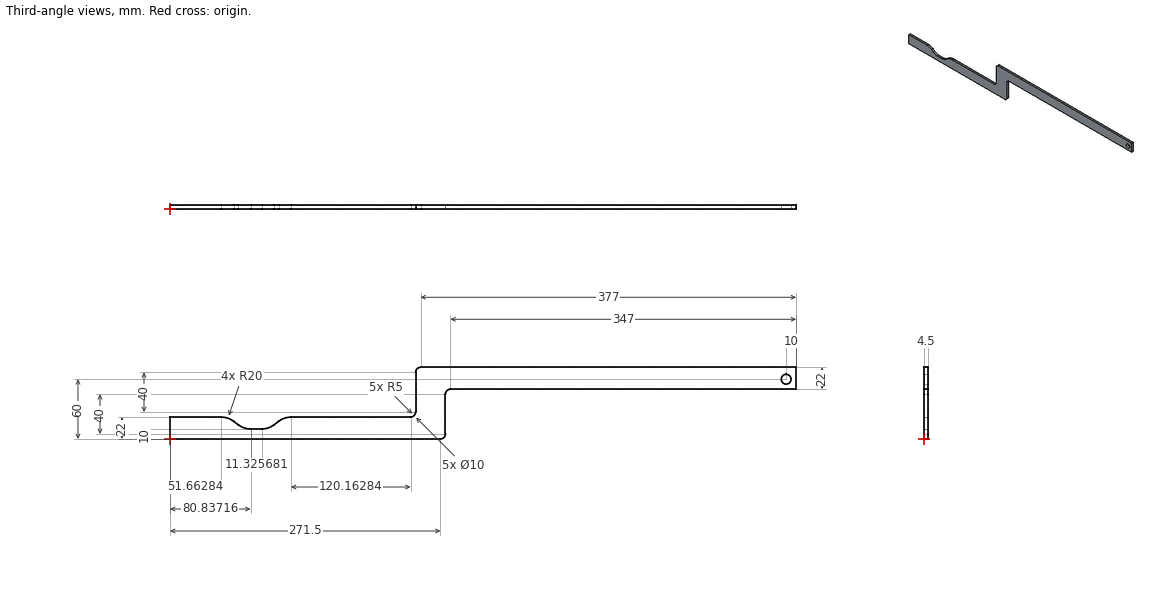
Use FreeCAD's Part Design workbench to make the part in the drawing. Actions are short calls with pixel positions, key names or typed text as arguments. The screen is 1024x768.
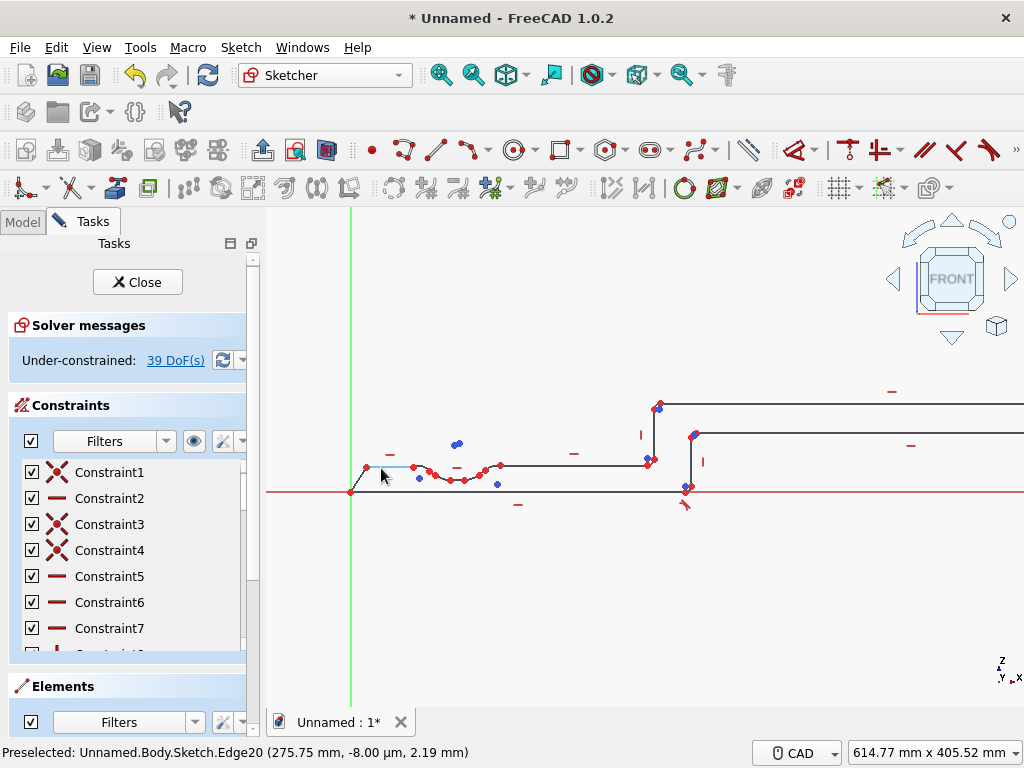
click(381, 467)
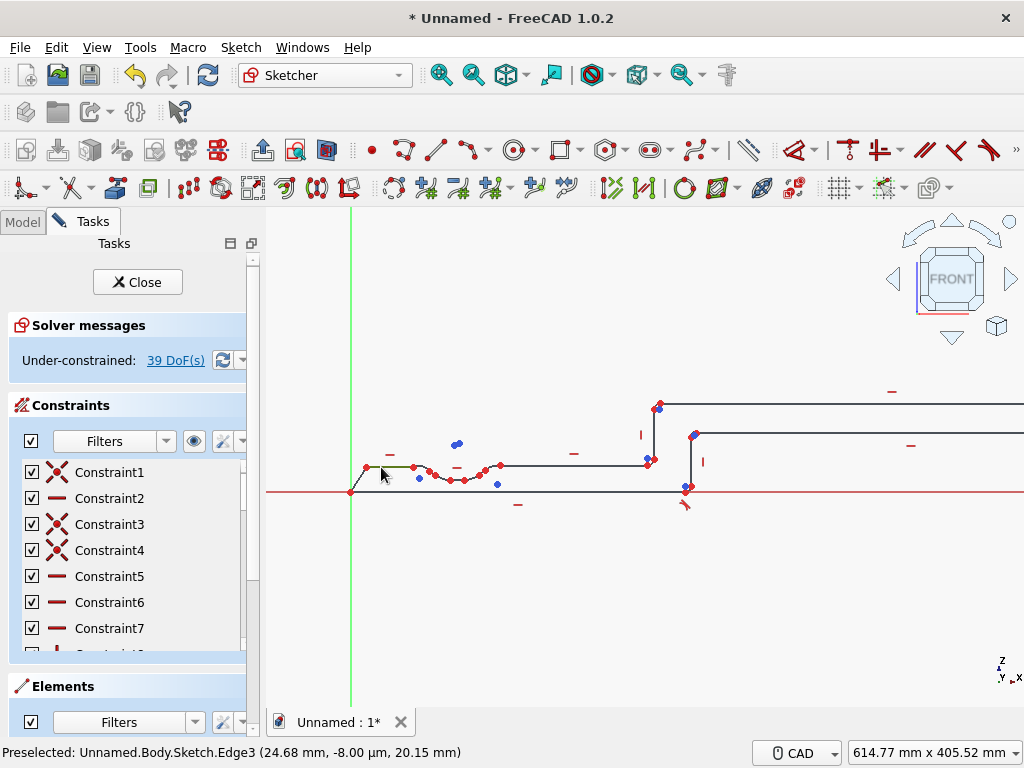
scroll(422, 466, up, 3)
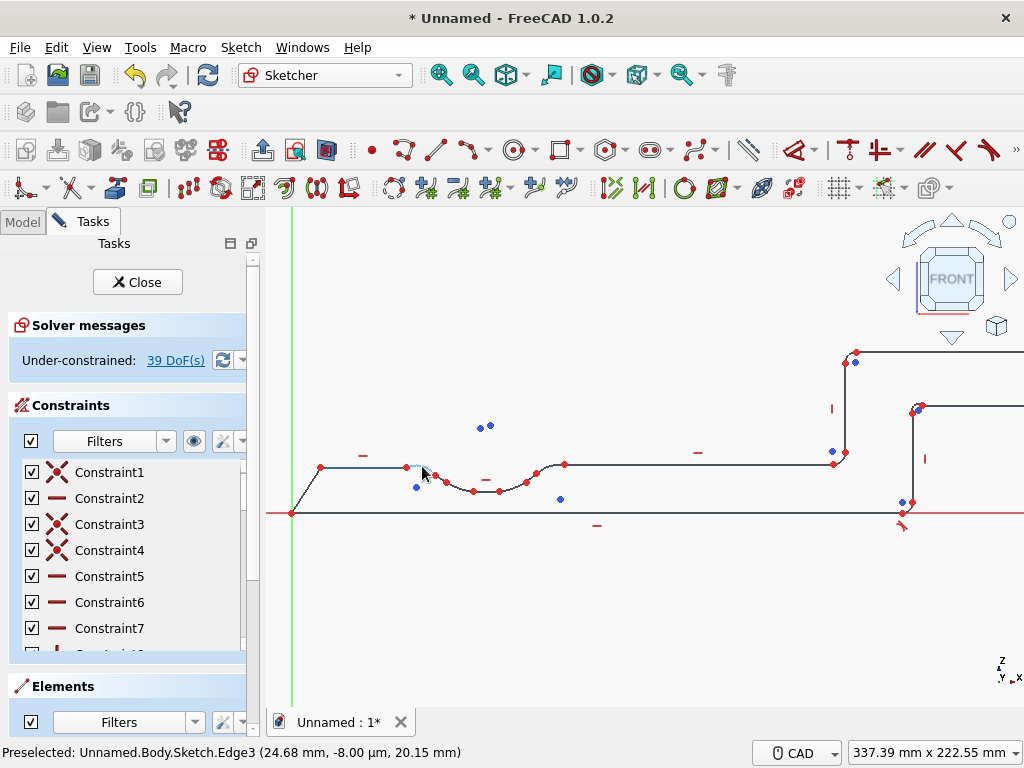
click(422, 466)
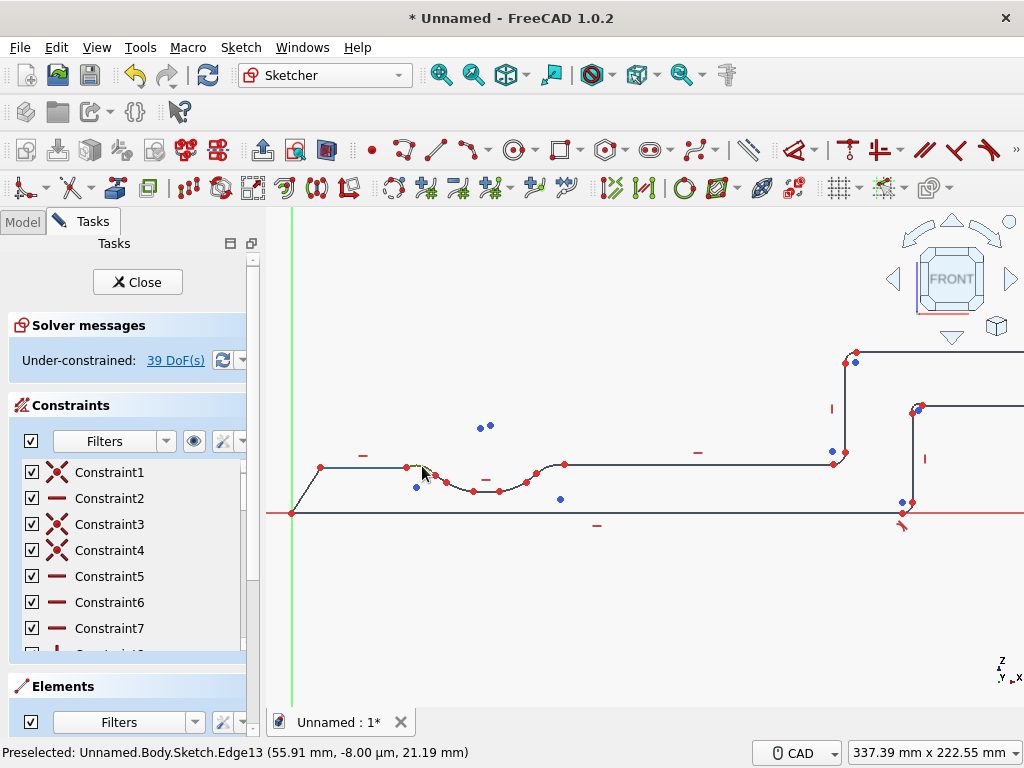
key(t)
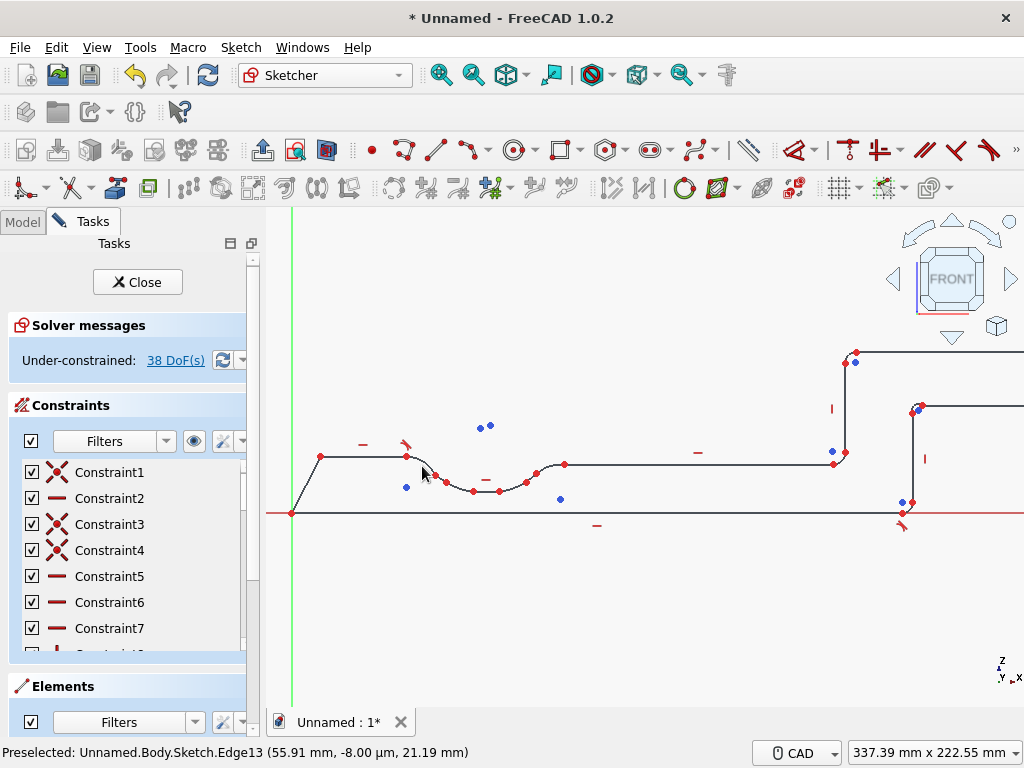
scroll(441, 479, up, 4)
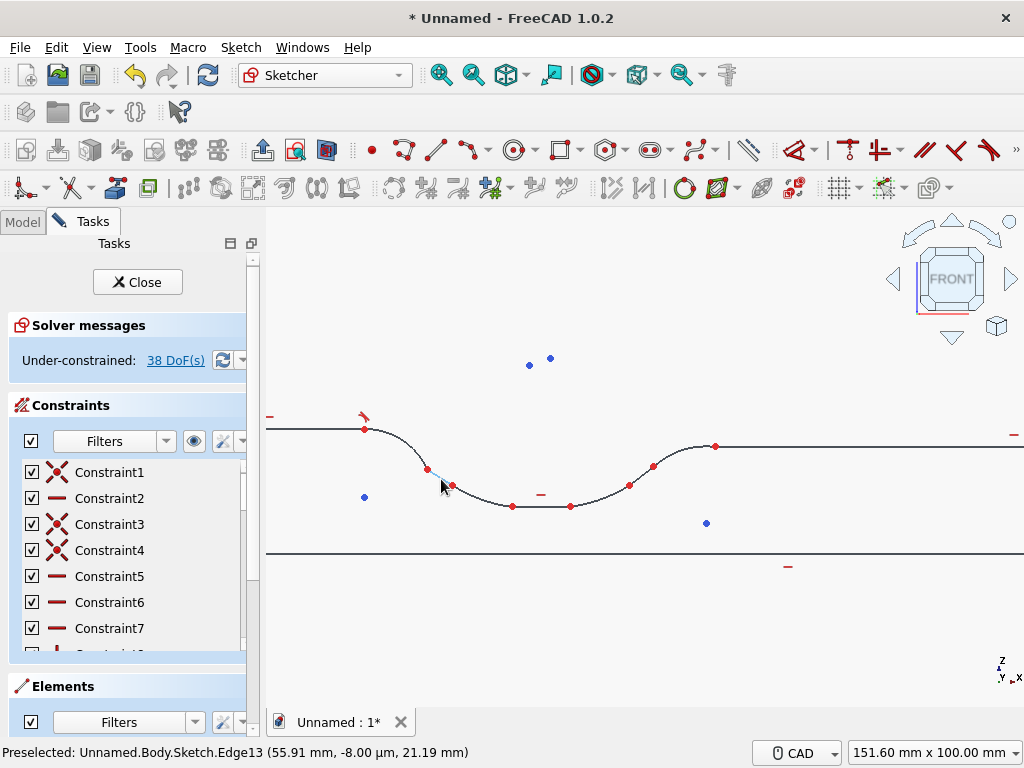
click(440, 478)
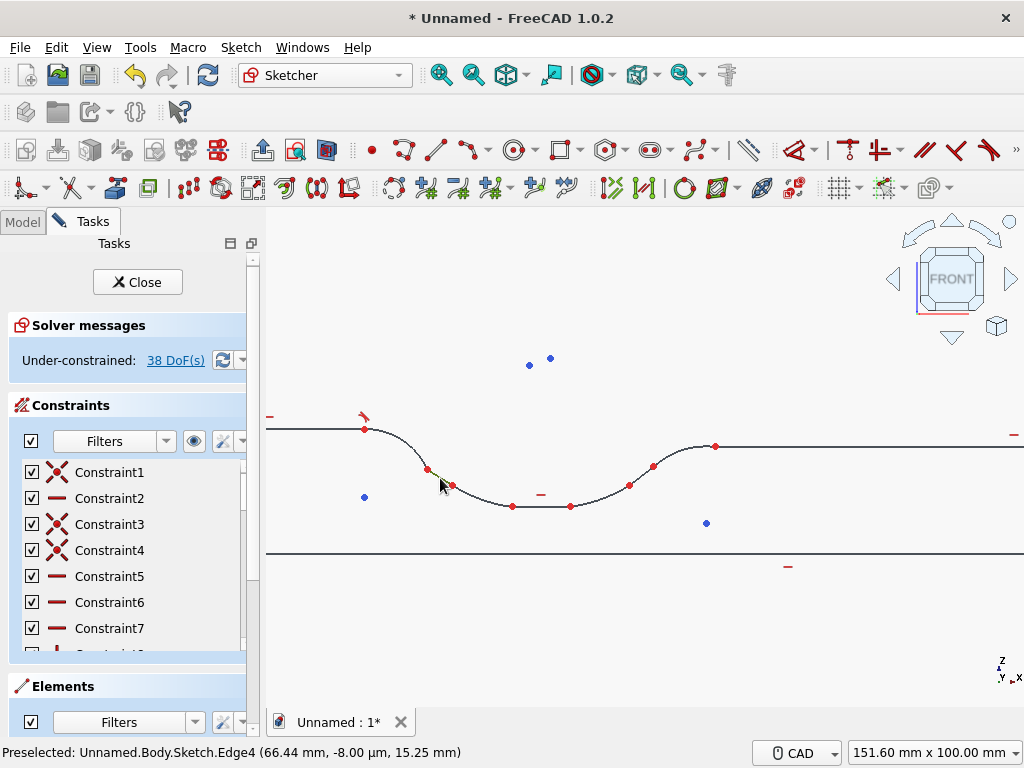
click(414, 450)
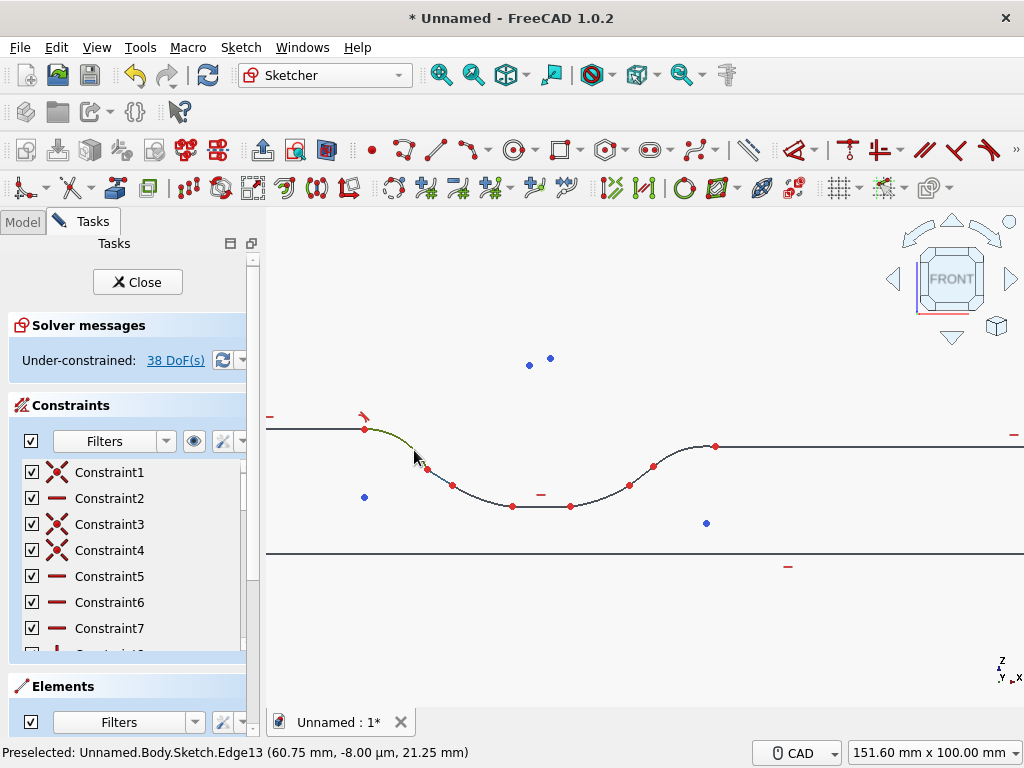
key(t)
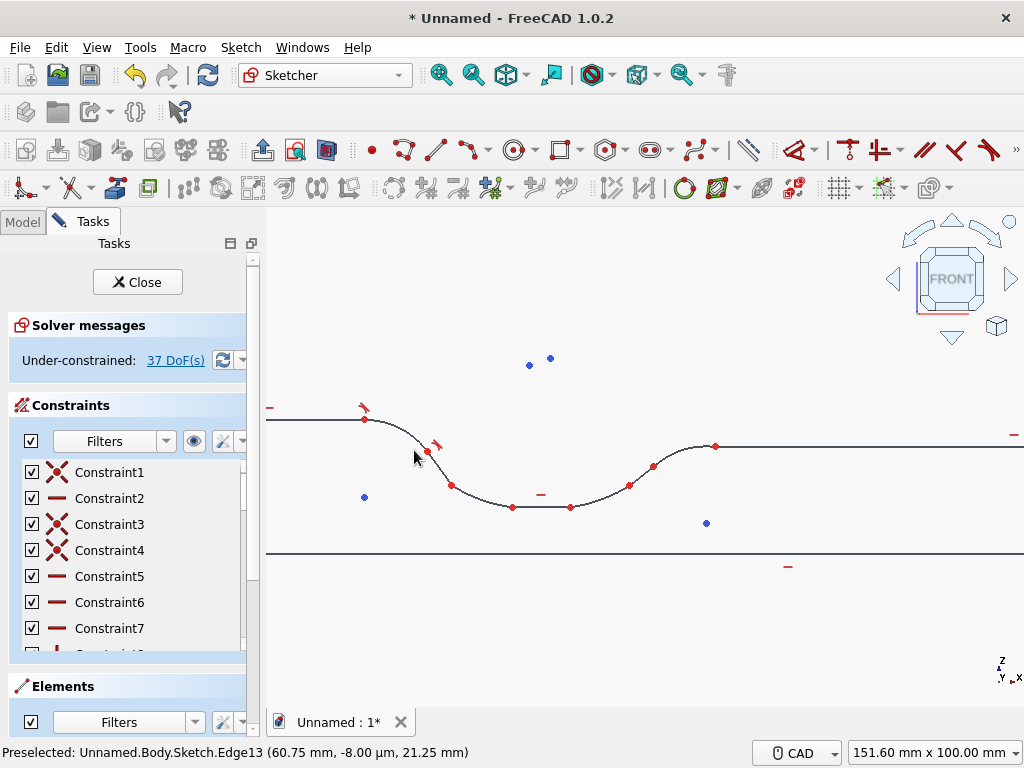
click(435, 462)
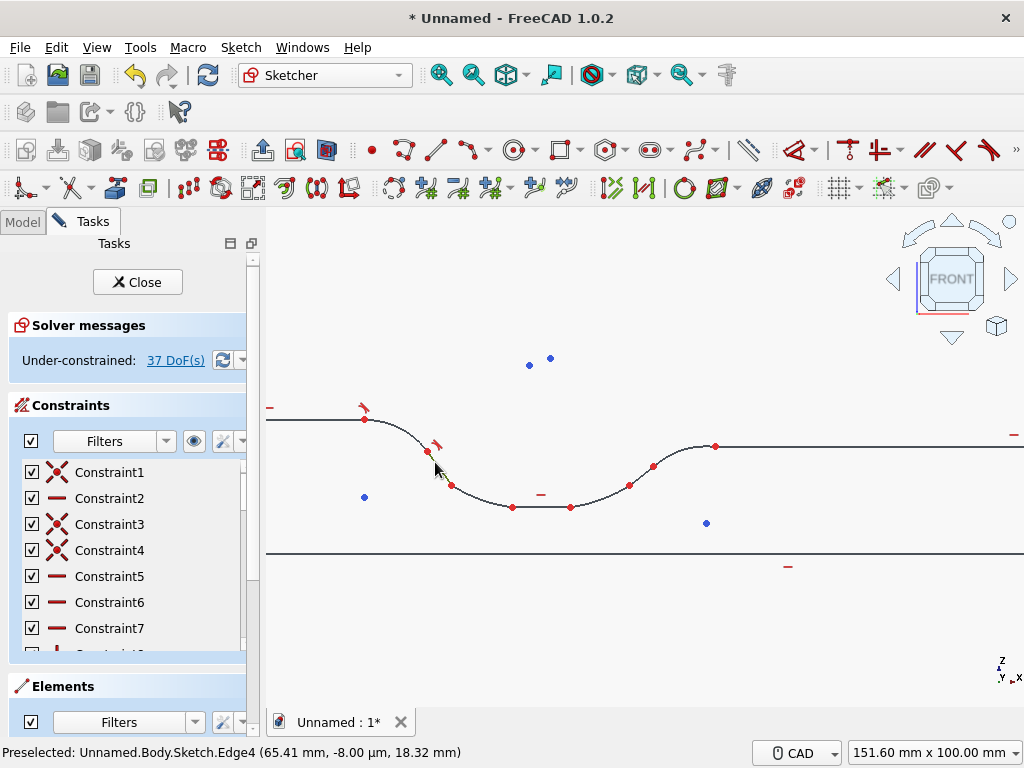
click(469, 495)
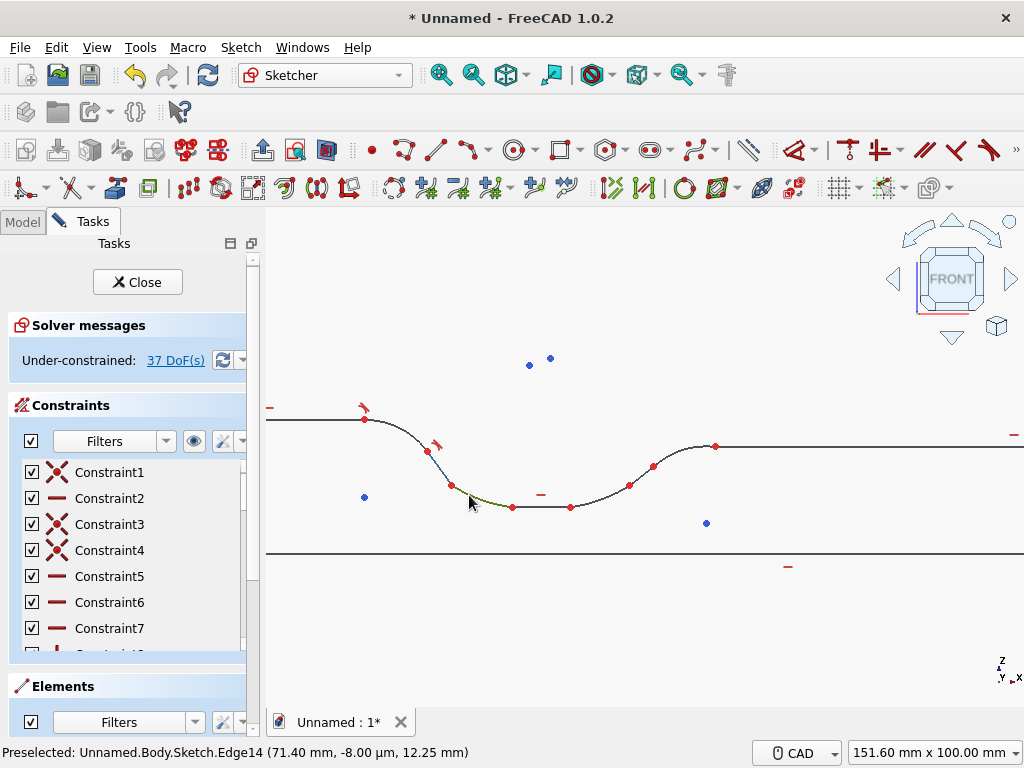
key(t)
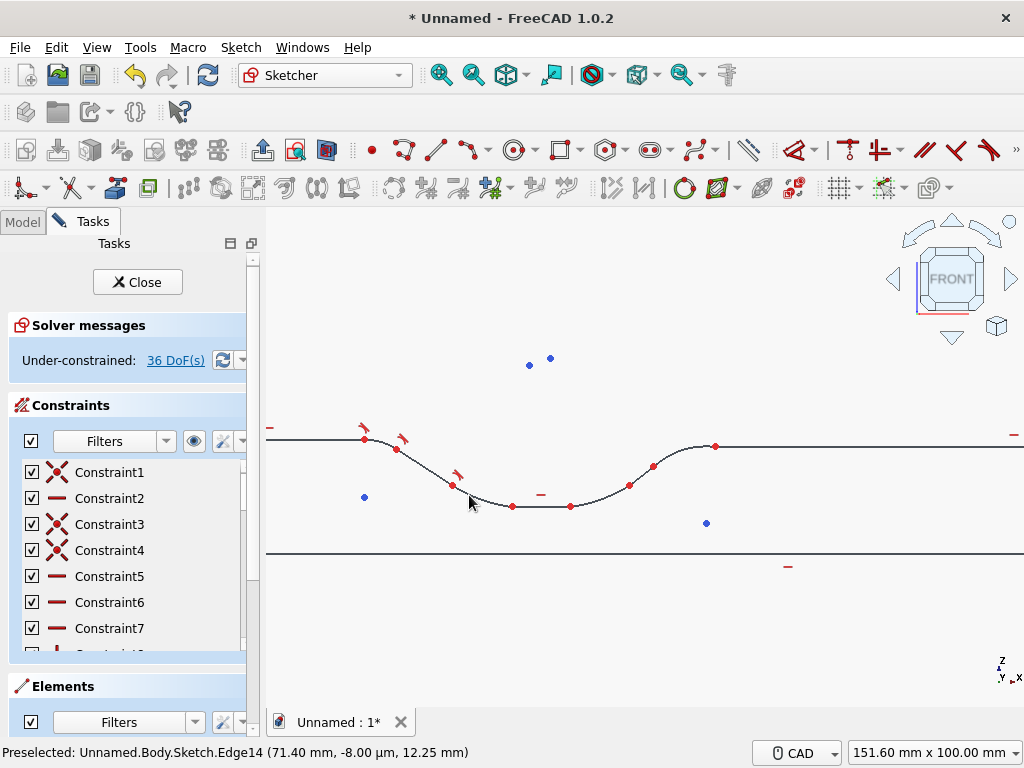
click(529, 507)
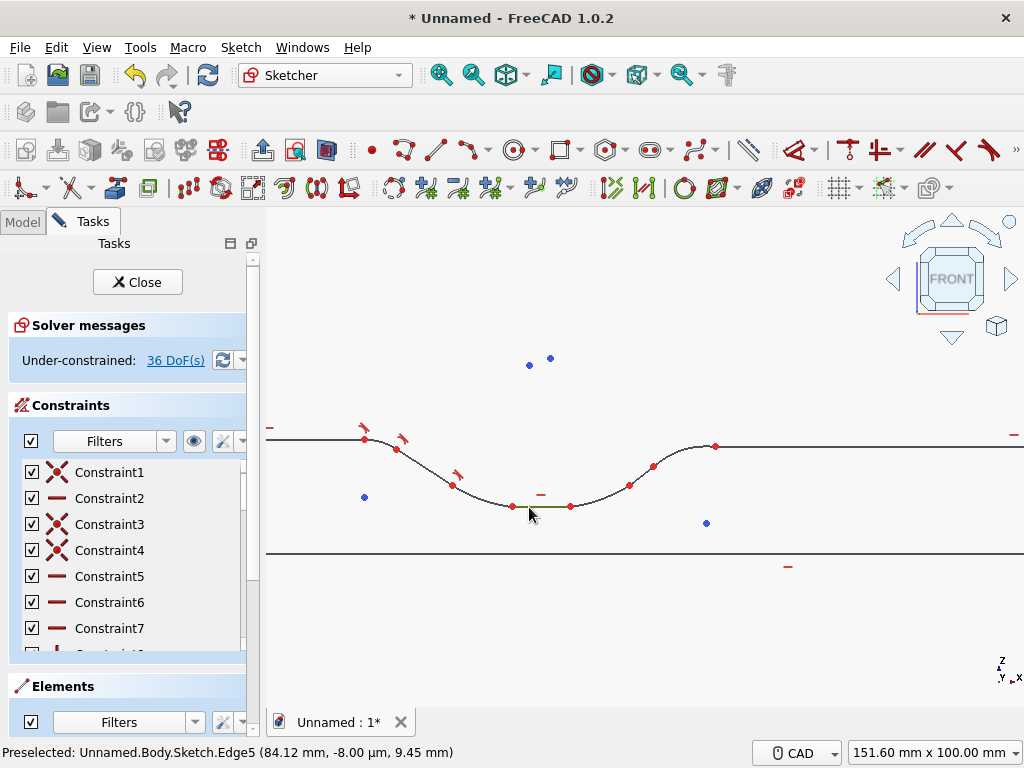
click(469, 495)